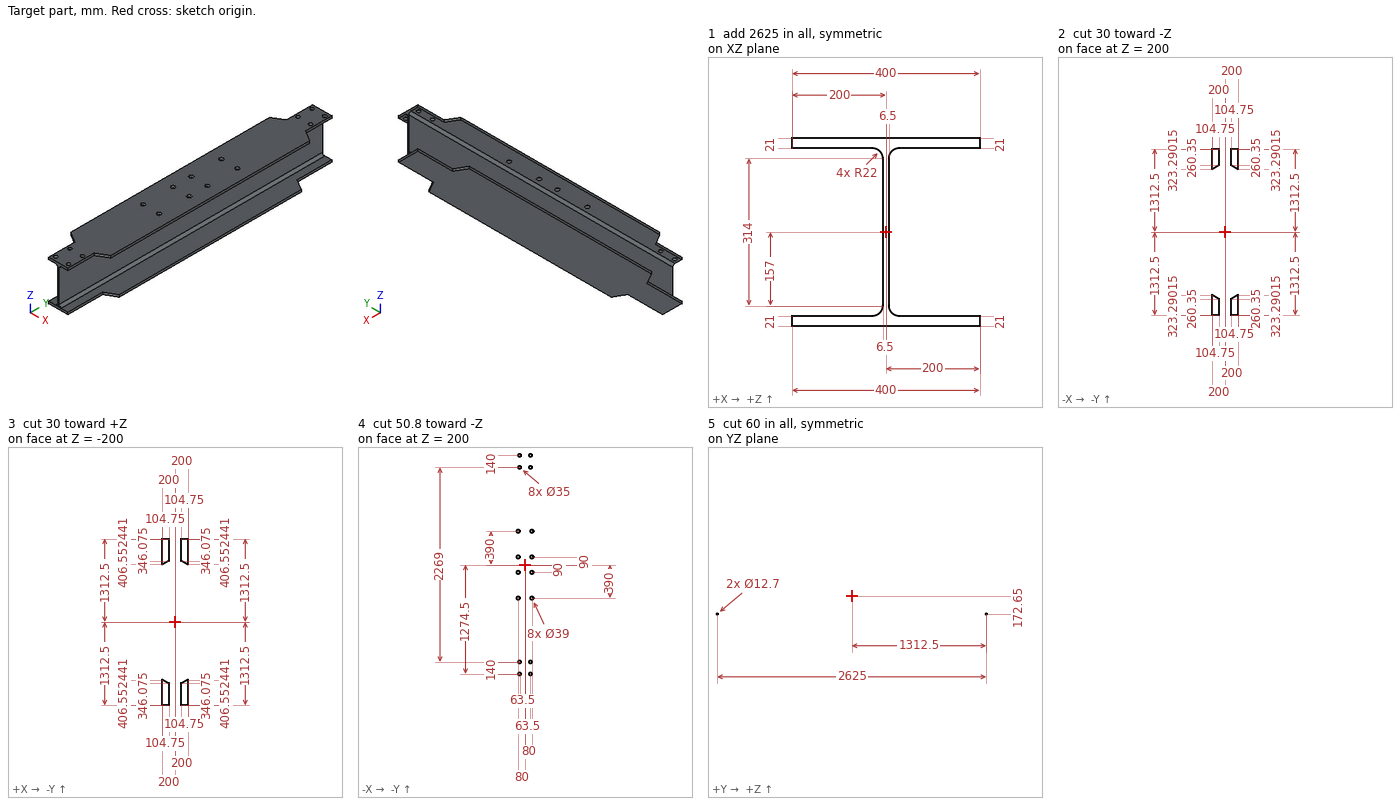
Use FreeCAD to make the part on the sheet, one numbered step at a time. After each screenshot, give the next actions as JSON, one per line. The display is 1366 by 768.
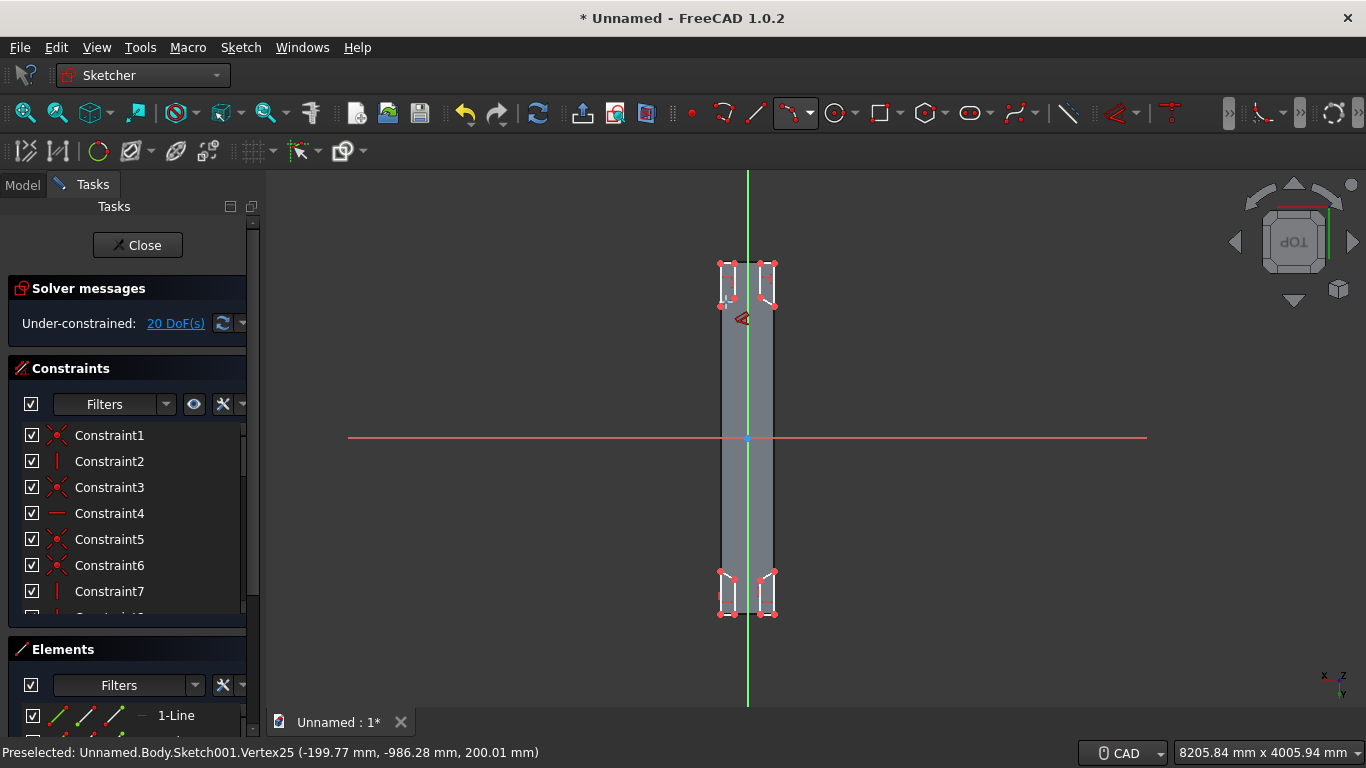
{"action": "scroll", "coordinate": [774, 572], "scroll_direction": "up", "scroll_amount": 2}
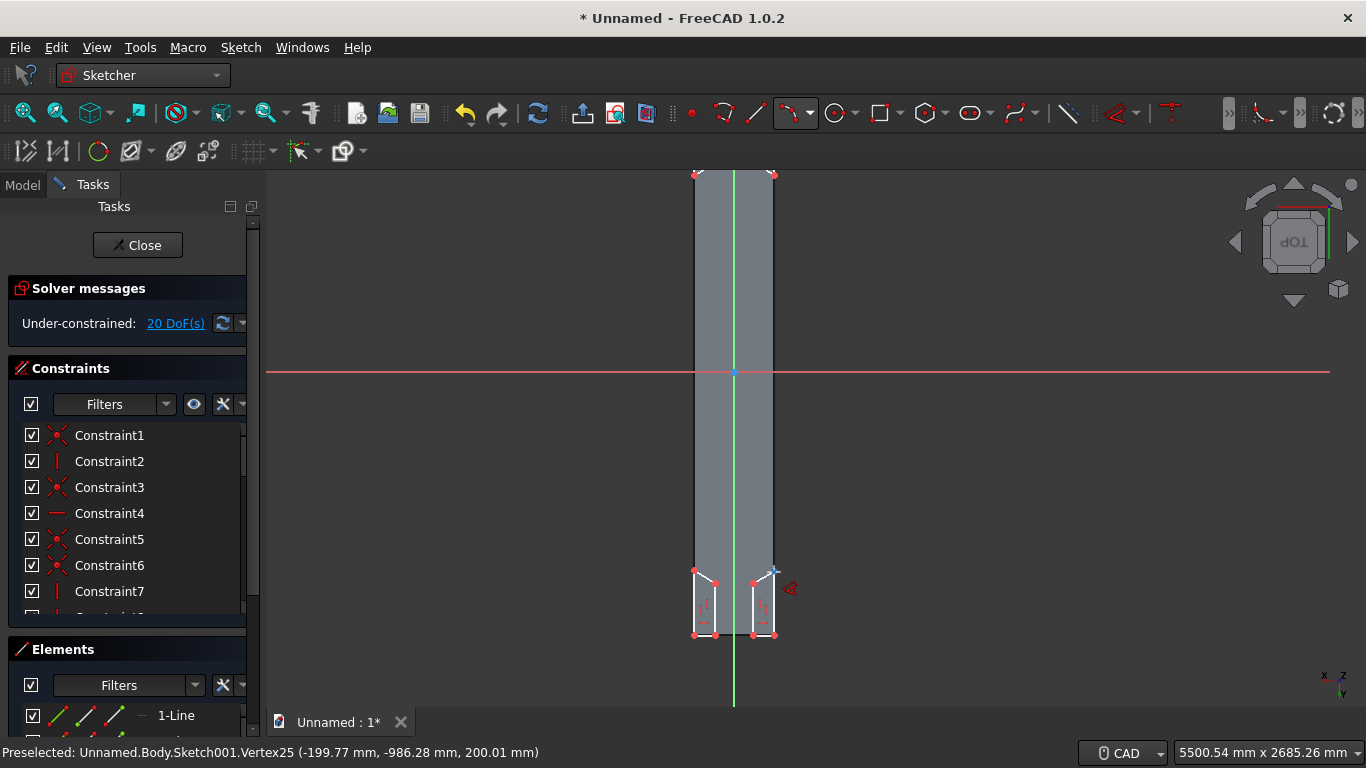
{"action": "left_click", "coordinate": [774, 571]}
{"action": "left_click", "coordinate": [754, 338]}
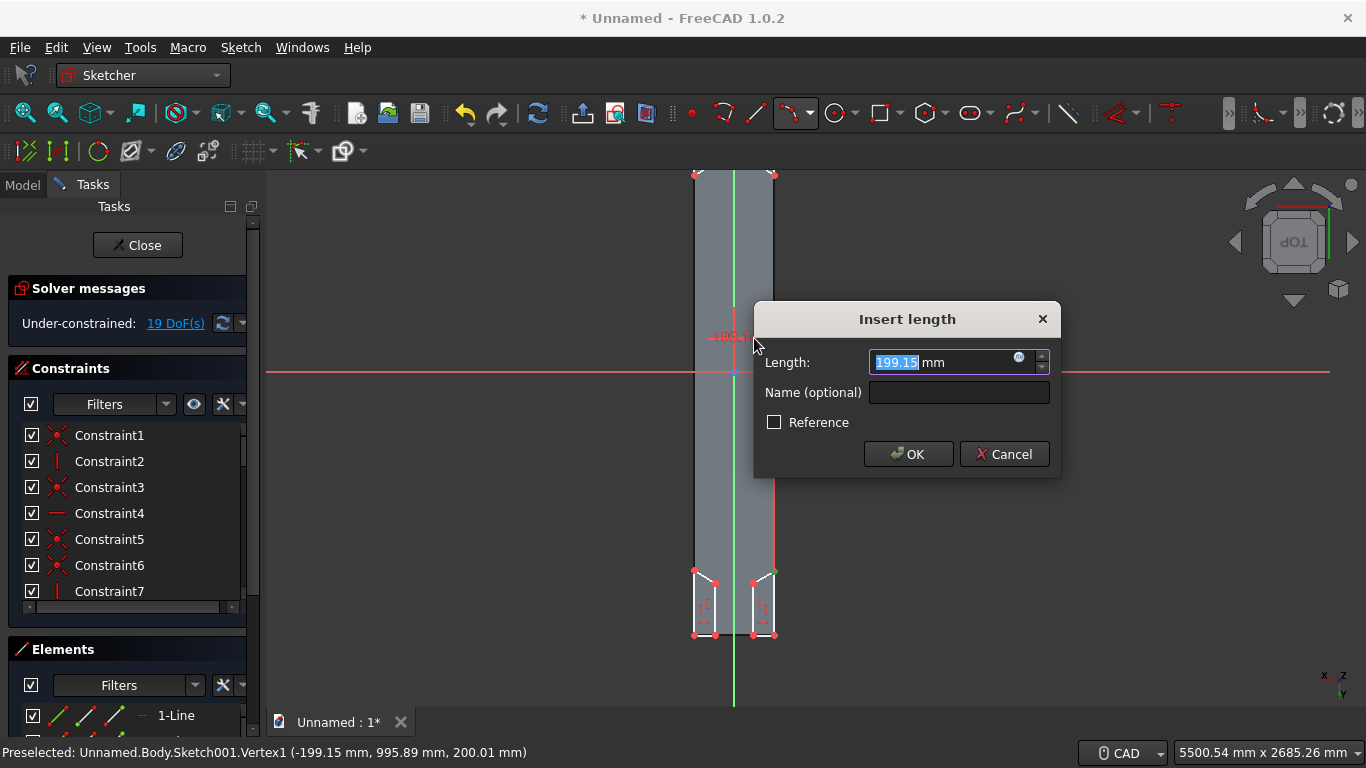
{"action": "type", "text": "200"}
{"action": "key", "text": "Return"}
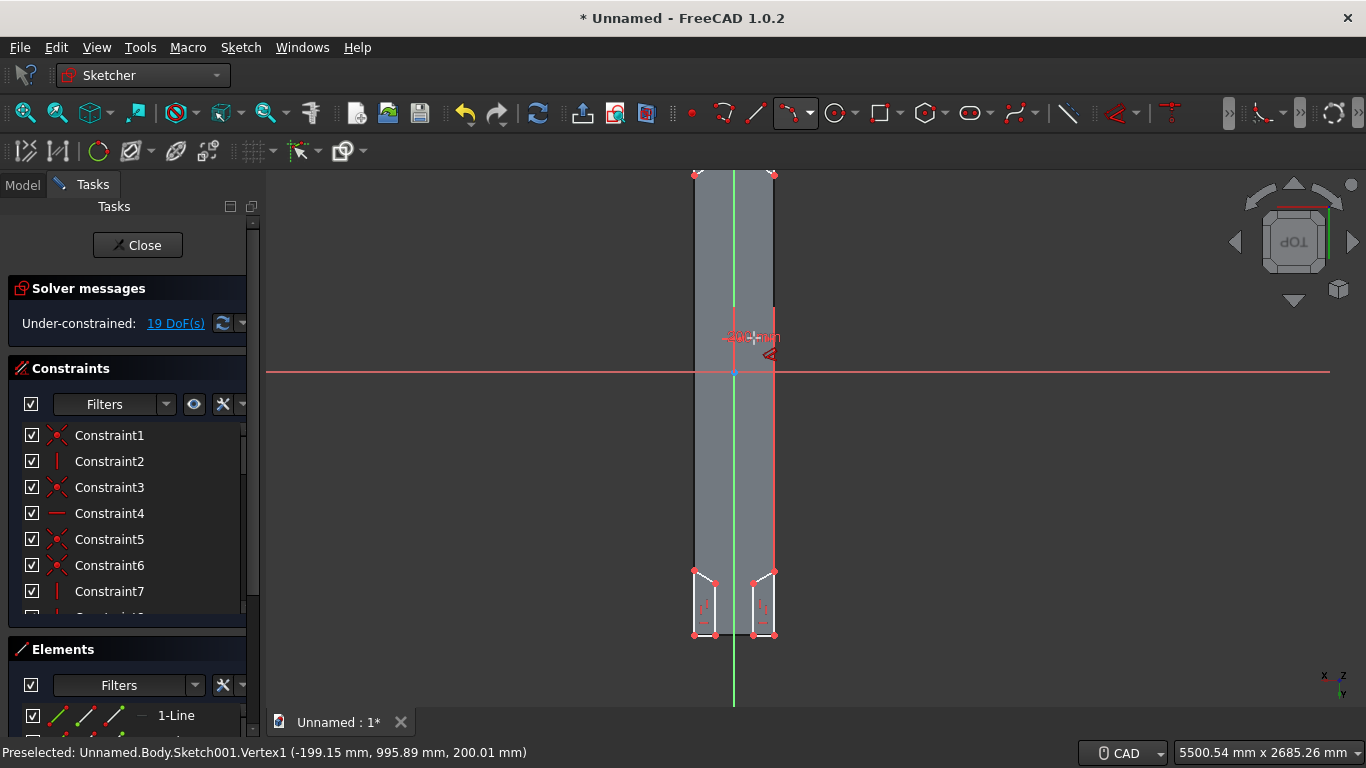
{"action": "left_click", "coordinate": [694, 571]}
{"action": "left_click", "coordinate": [714, 314]}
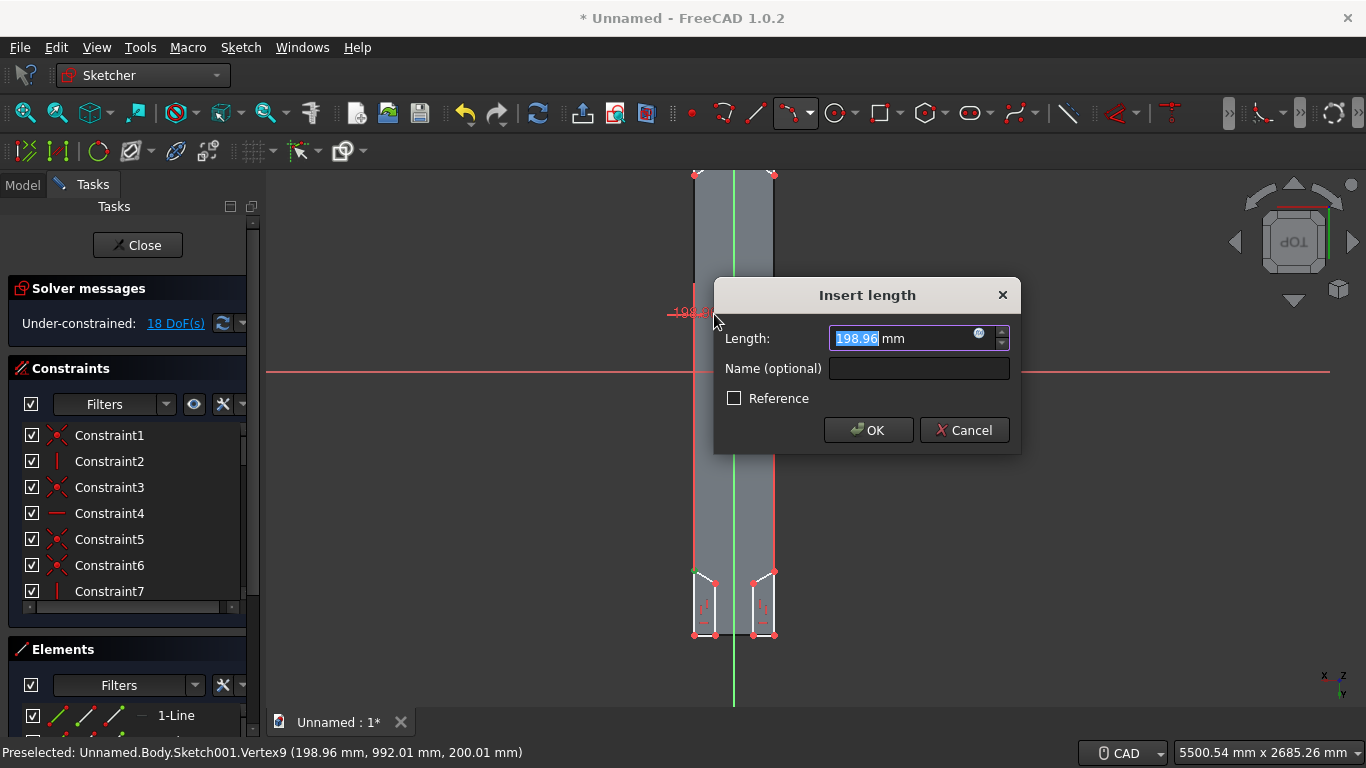
{"action": "type", "text": "200"}
{"action": "key", "text": "Return"}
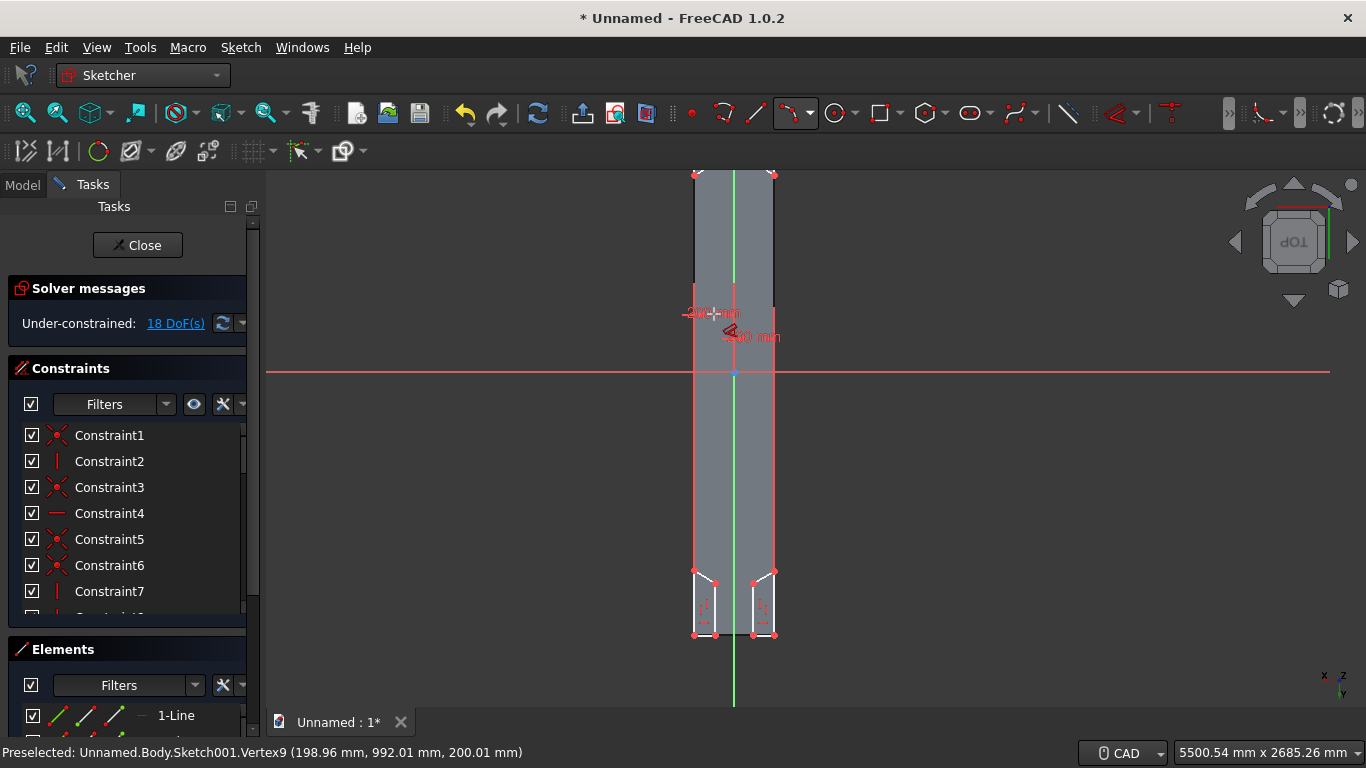
{"action": "scroll", "coordinate": [774, 573], "scroll_direction": "down", "scroll_amount": 2}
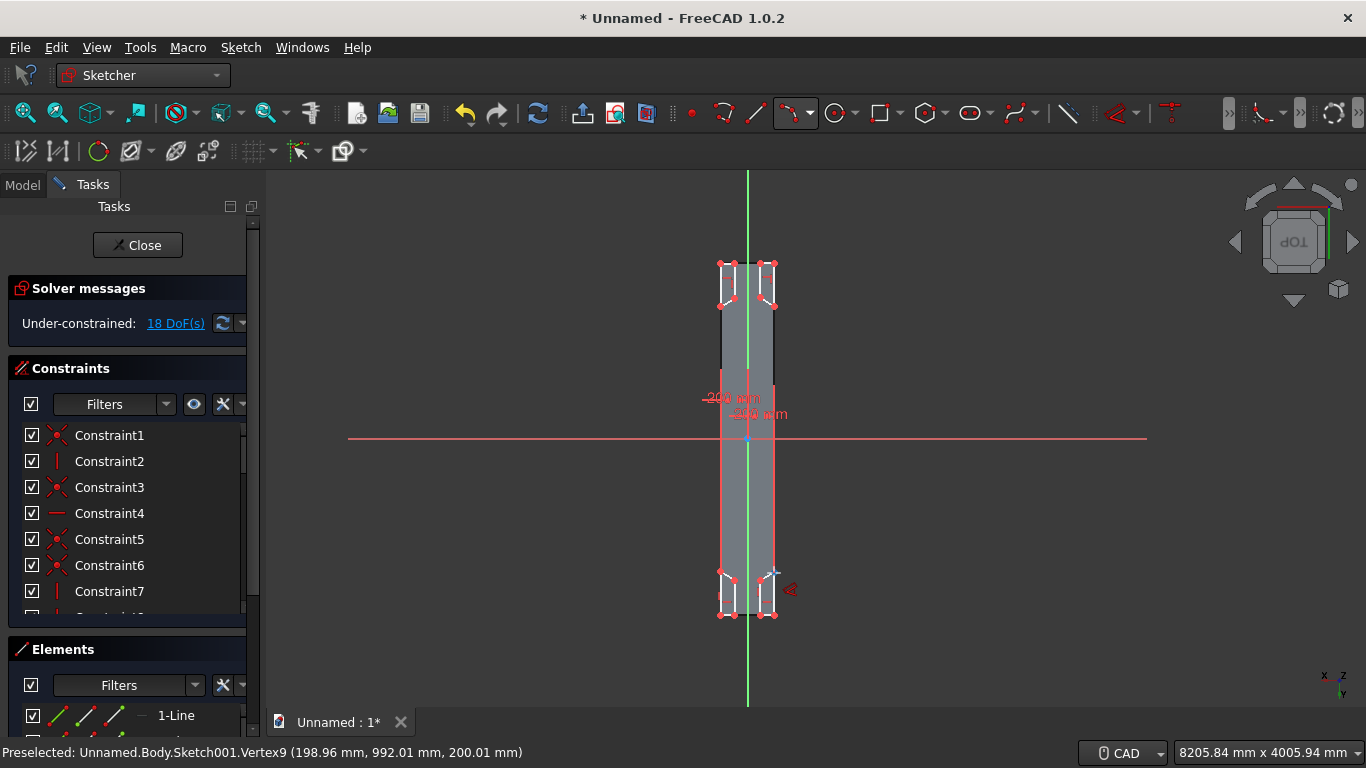
{"action": "scroll", "coordinate": [721, 307], "scroll_direction": "up", "scroll_amount": 2}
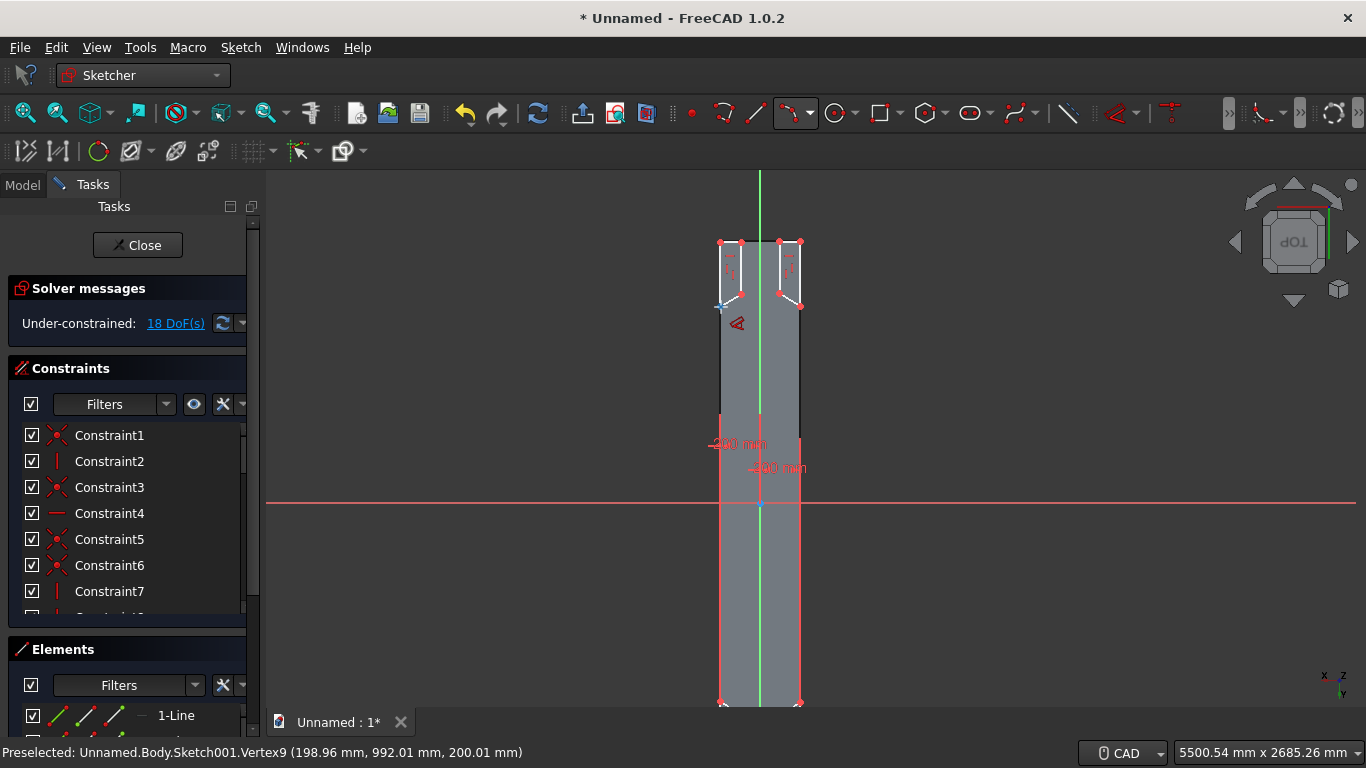
{"action": "left_click", "coordinate": [720, 307]}
{"action": "left_click", "coordinate": [740, 537]}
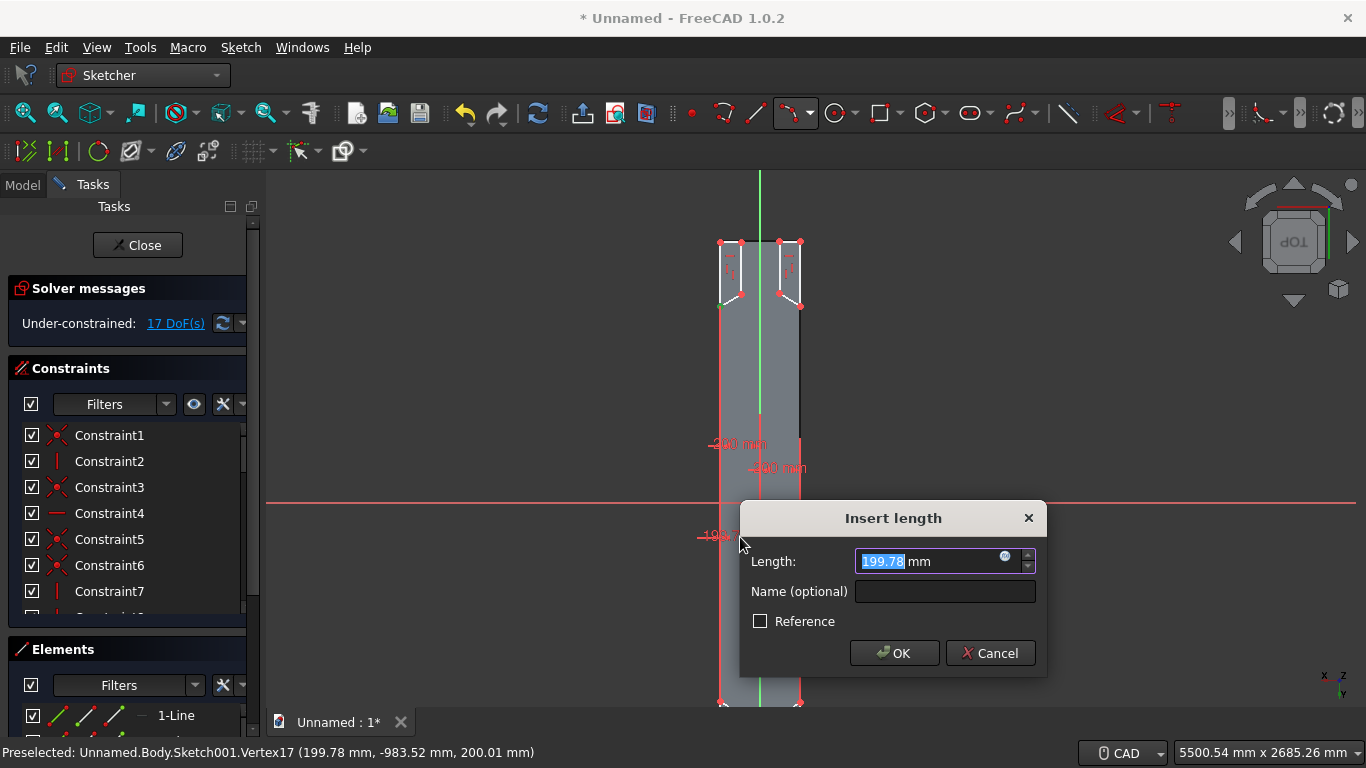
{"action": "type", "text": "200"}
{"action": "key", "text": "Return"}